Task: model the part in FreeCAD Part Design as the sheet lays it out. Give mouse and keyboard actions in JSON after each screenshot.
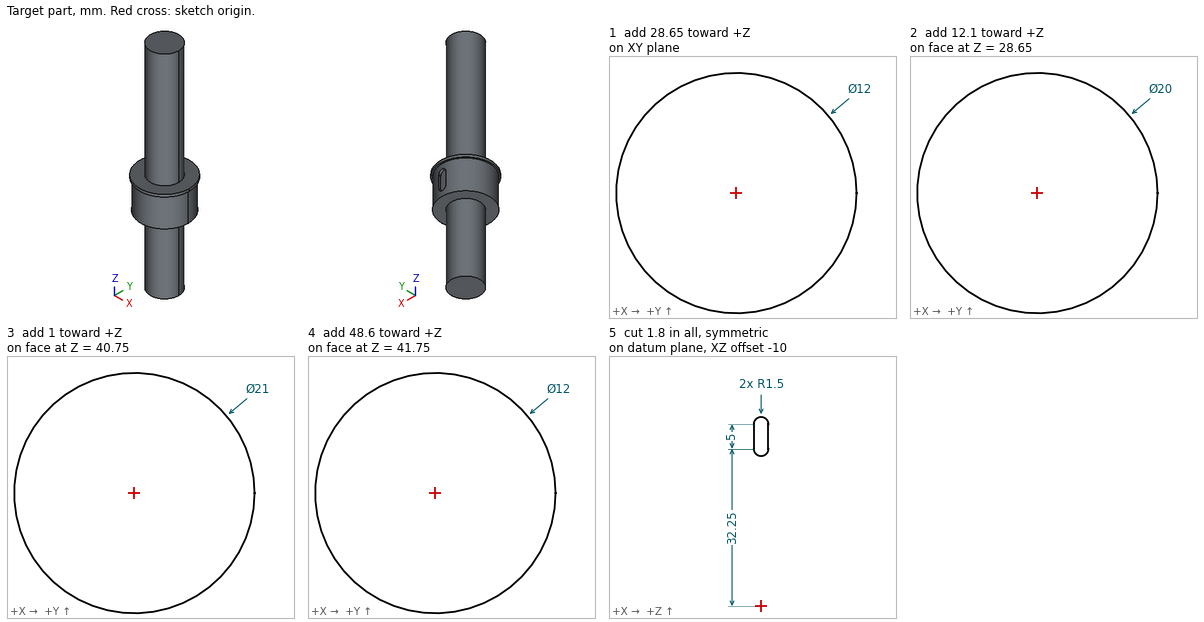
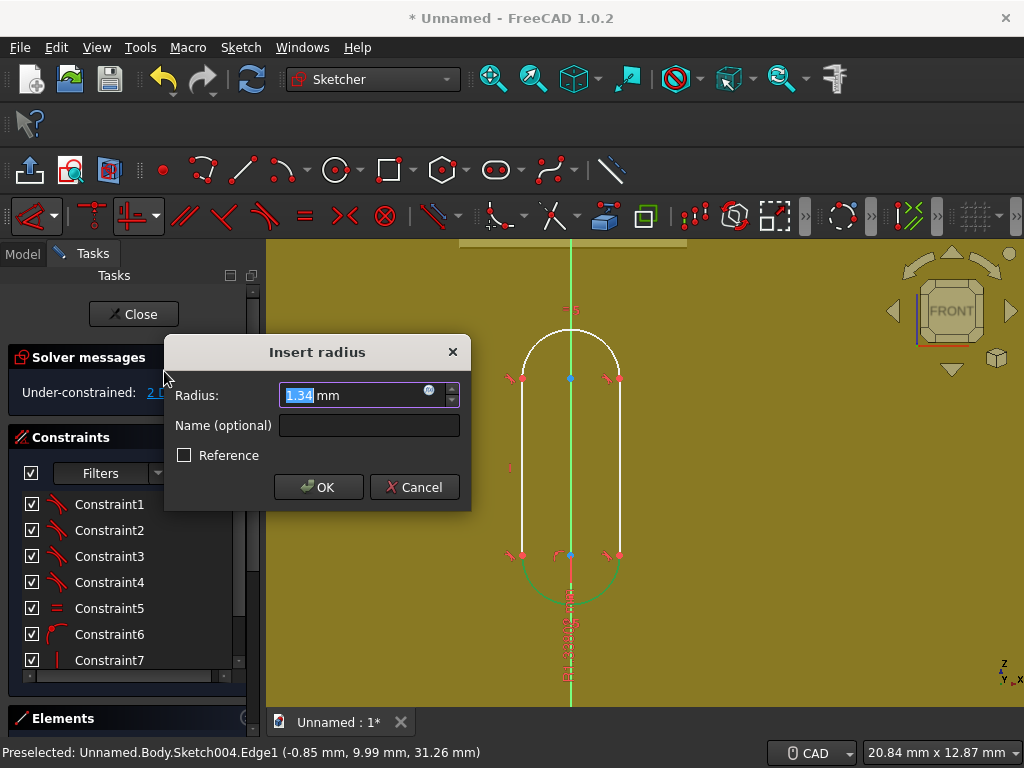
{"action": "type", "text": "1.5"}
{"action": "key", "text": "Return"}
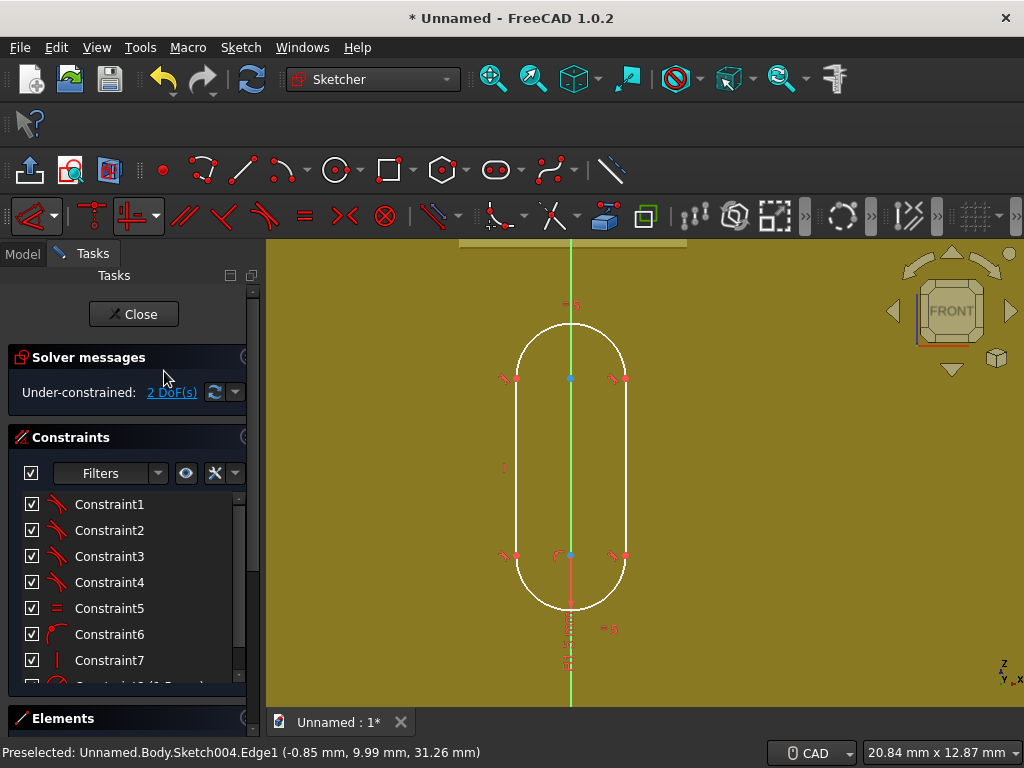
{"action": "left_click", "coordinate": [516, 503]}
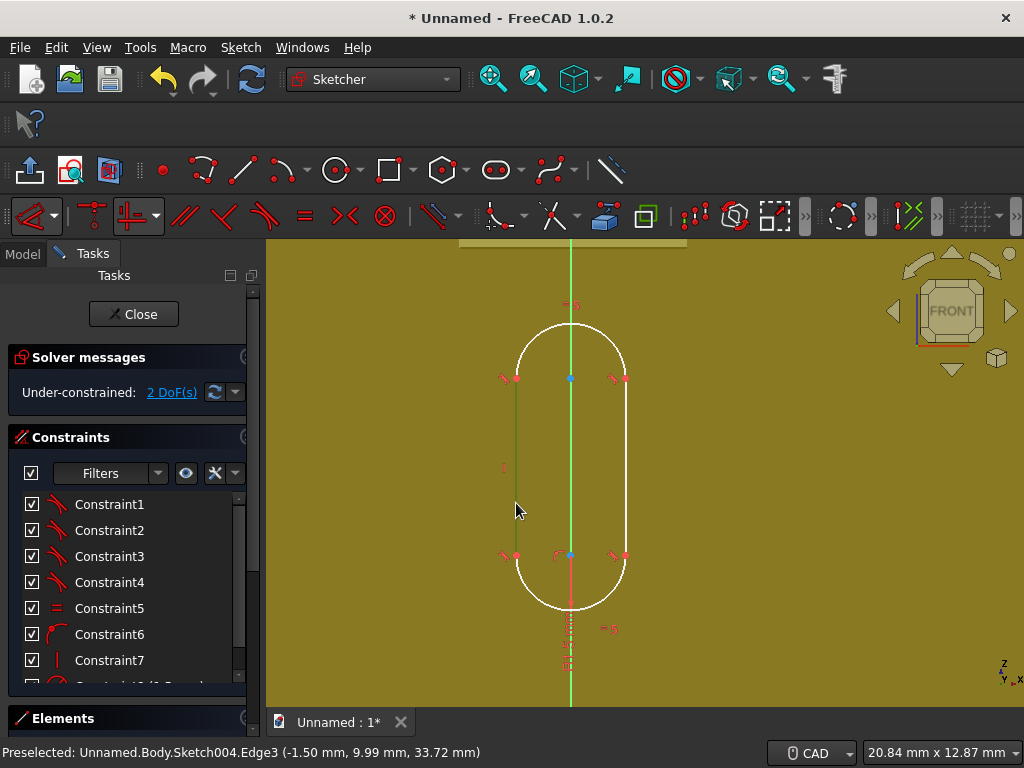
{"action": "key", "text": "i"}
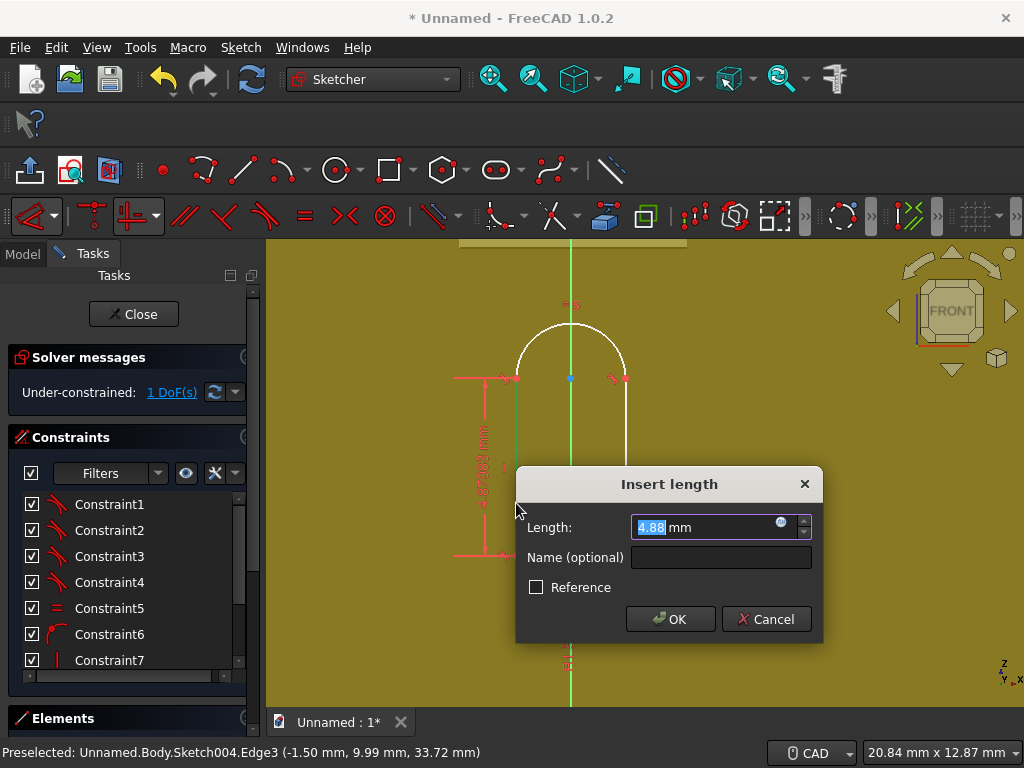
{"action": "type", "text": "5"}
{"action": "key", "text": "Return"}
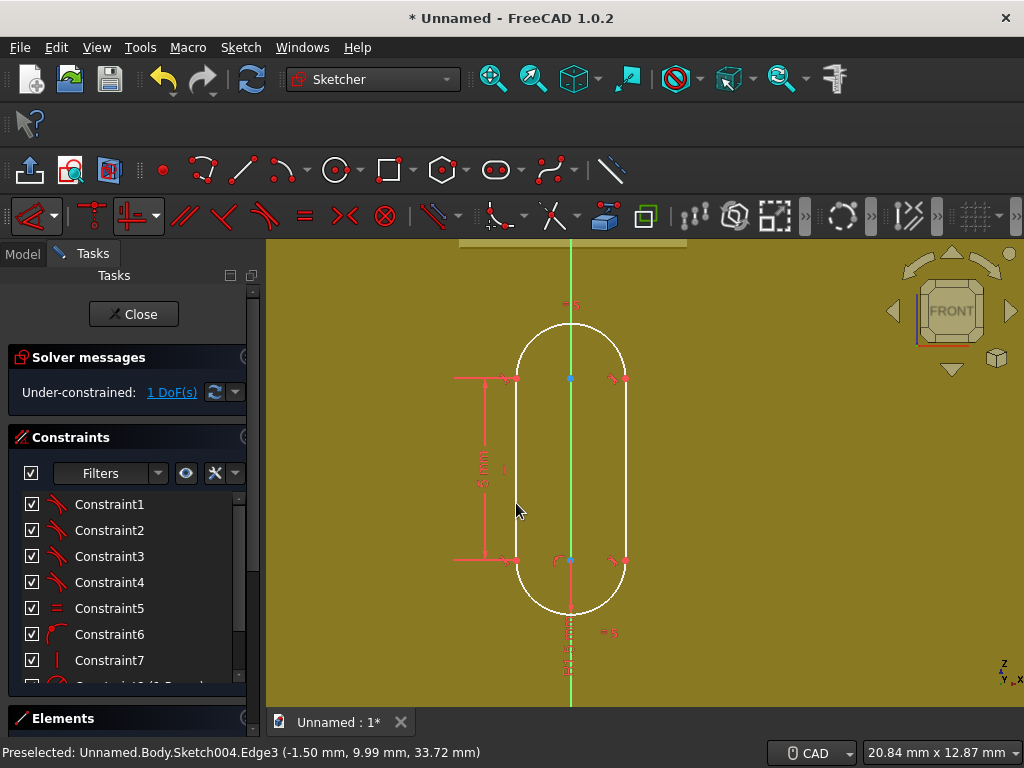
{"action": "left_click", "coordinate": [516, 560]}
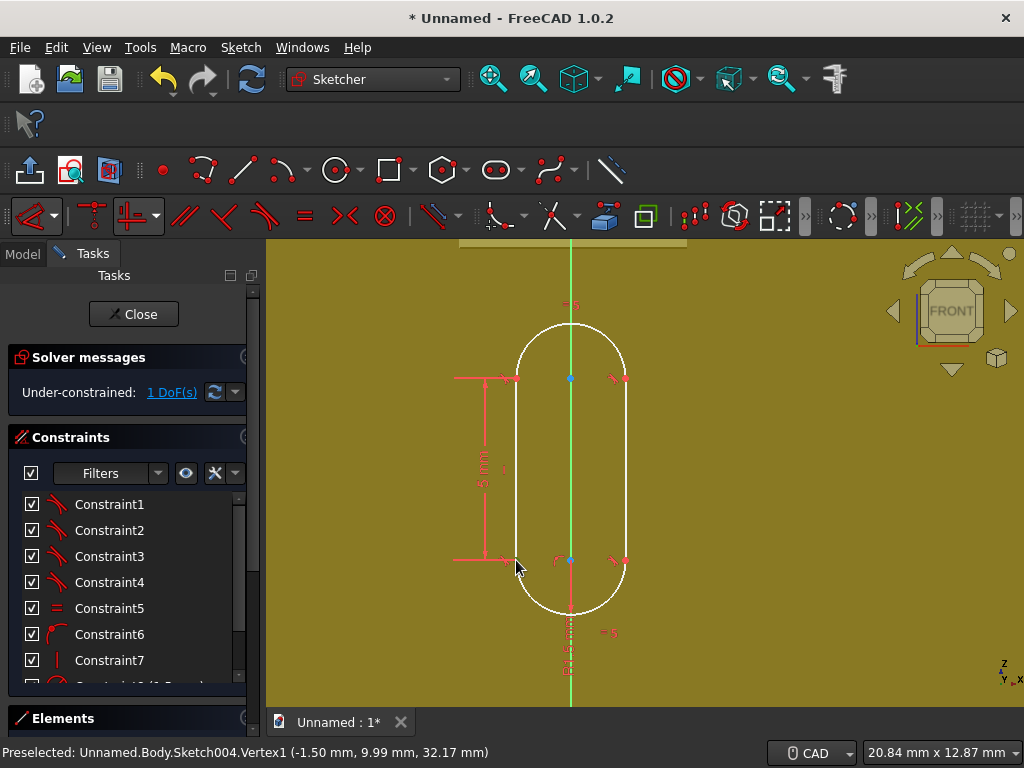
{"action": "left_click", "coordinate": [56, 216]}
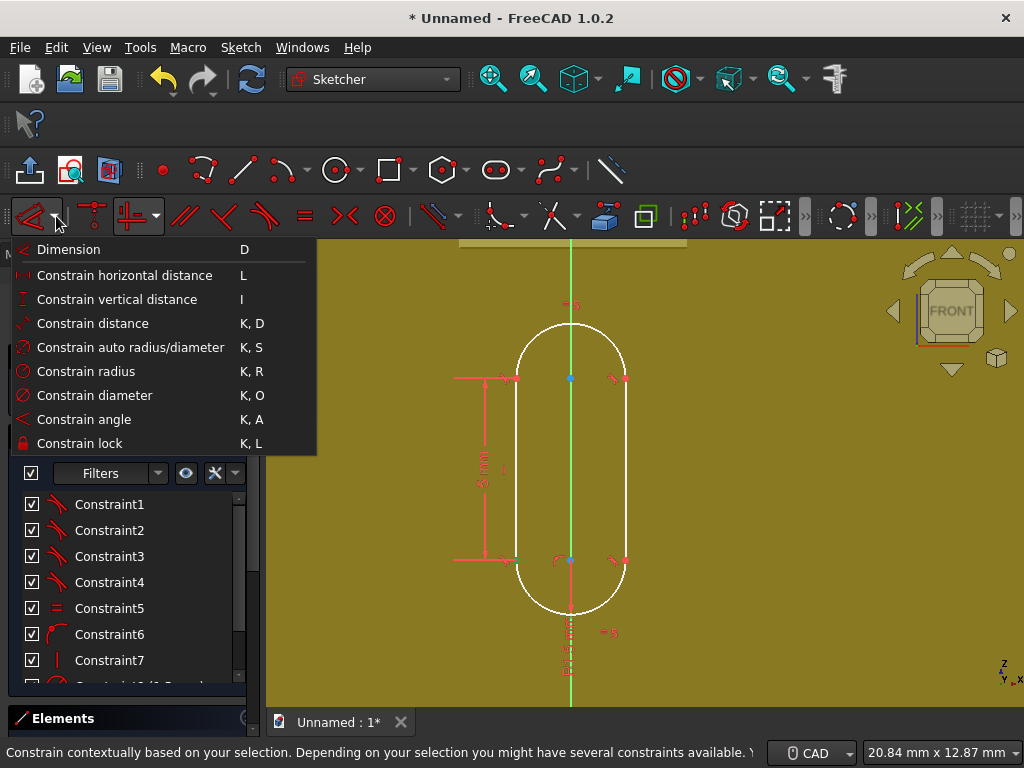
{"action": "left_click", "coordinate": [164, 299]}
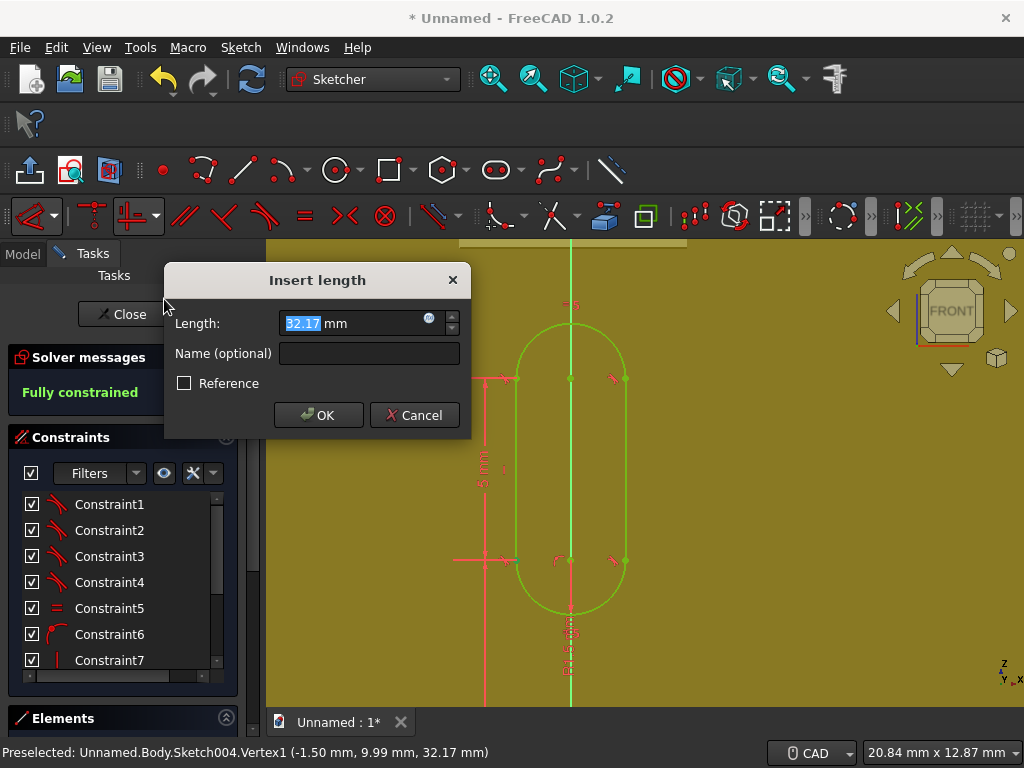
{"action": "type", "text": "32.25"}
{"action": "key", "text": "Return"}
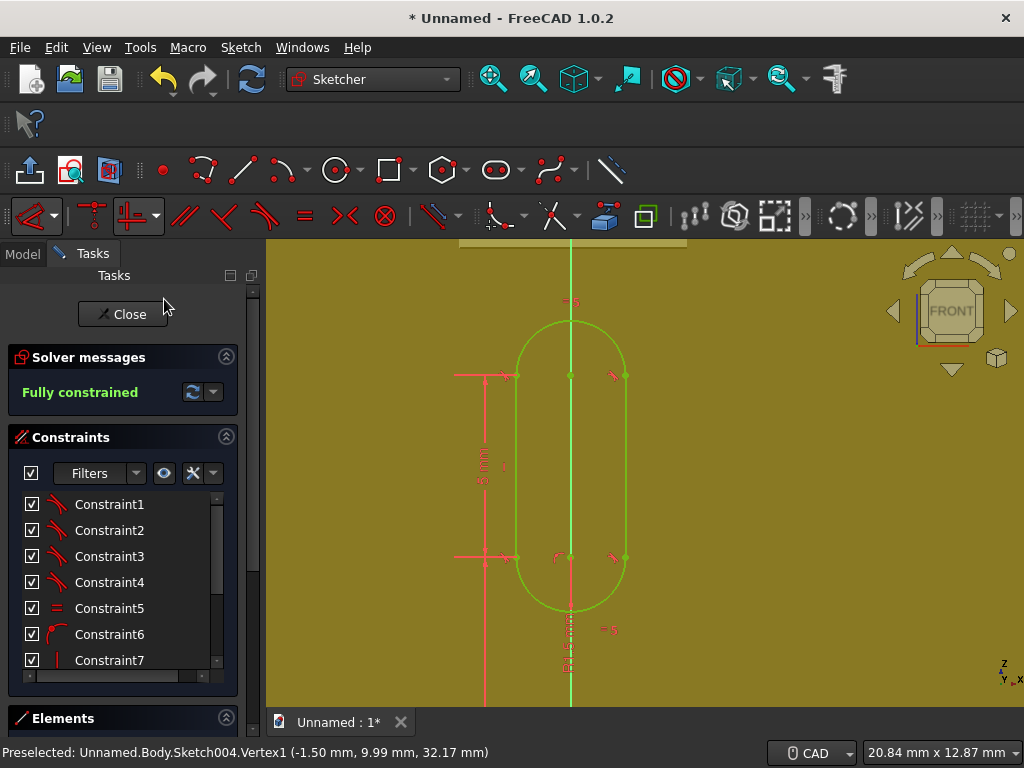
{"action": "left_click", "coordinate": [123, 314]}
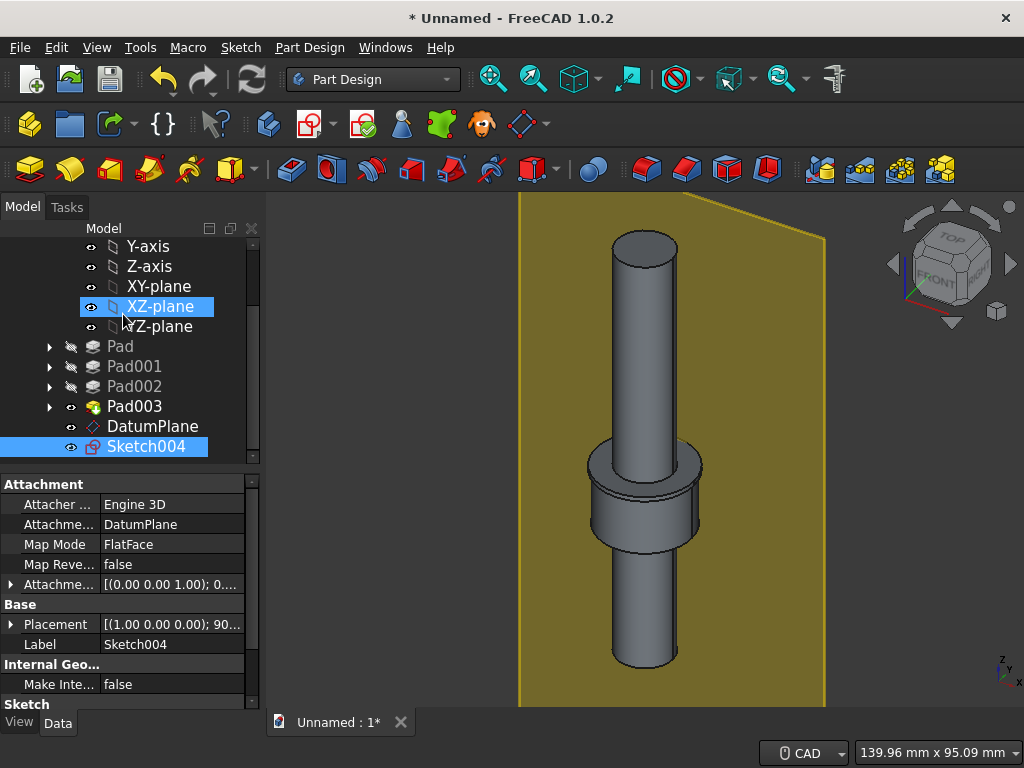
{"action": "left_click", "coordinate": [292, 170]}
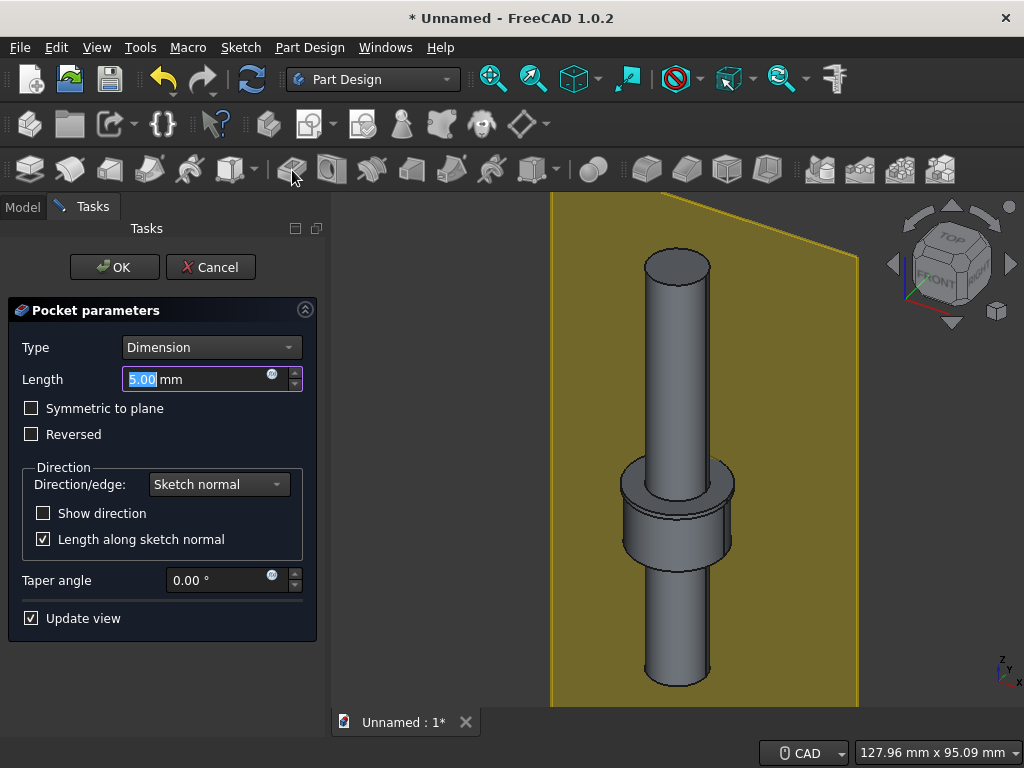
{"action": "type", "text": "1.8"}
{"action": "key", "text": "Tab"}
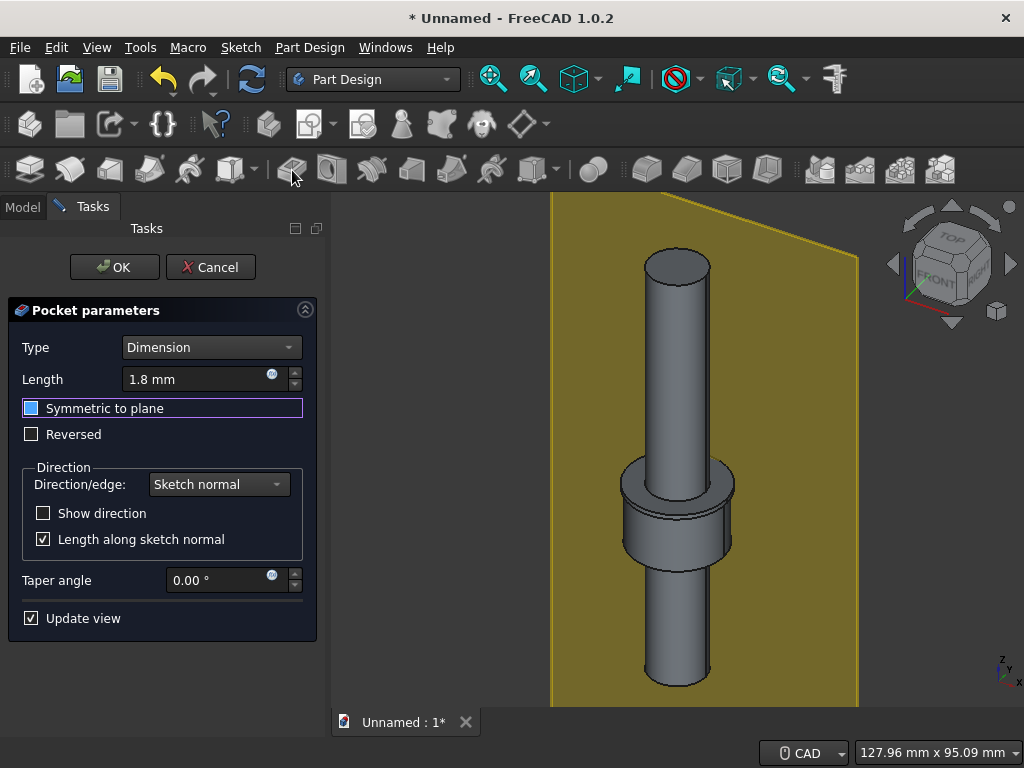
{"action": "left_click", "coordinate": [30, 408]}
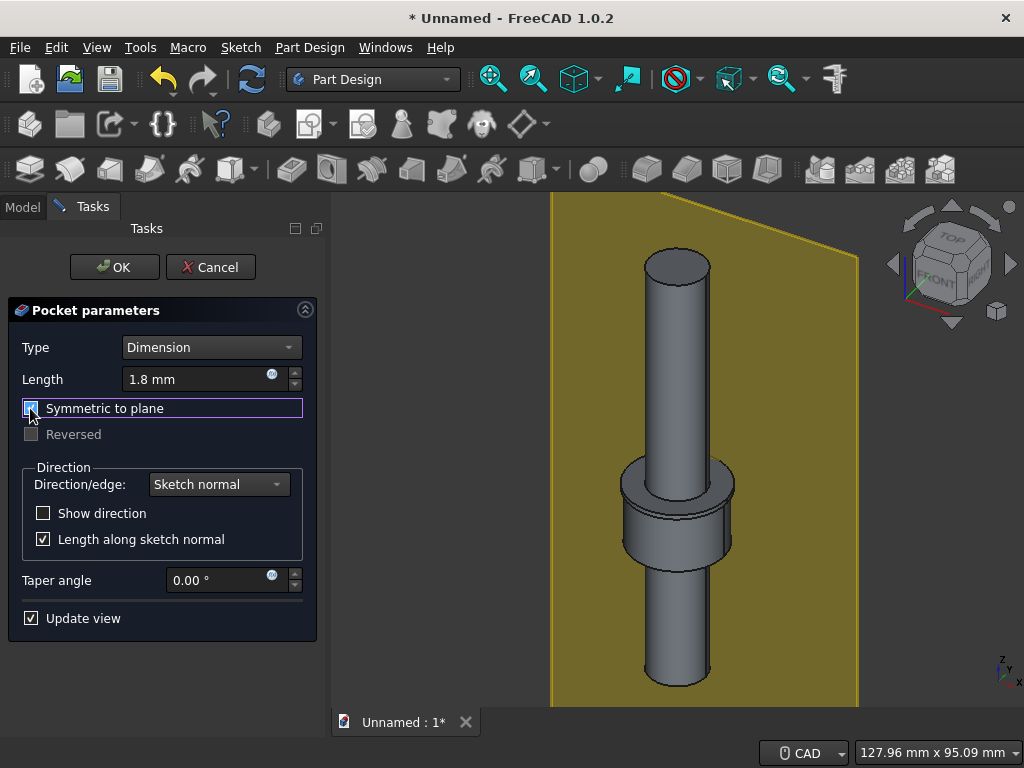
{"action": "left_click", "coordinate": [115, 267]}